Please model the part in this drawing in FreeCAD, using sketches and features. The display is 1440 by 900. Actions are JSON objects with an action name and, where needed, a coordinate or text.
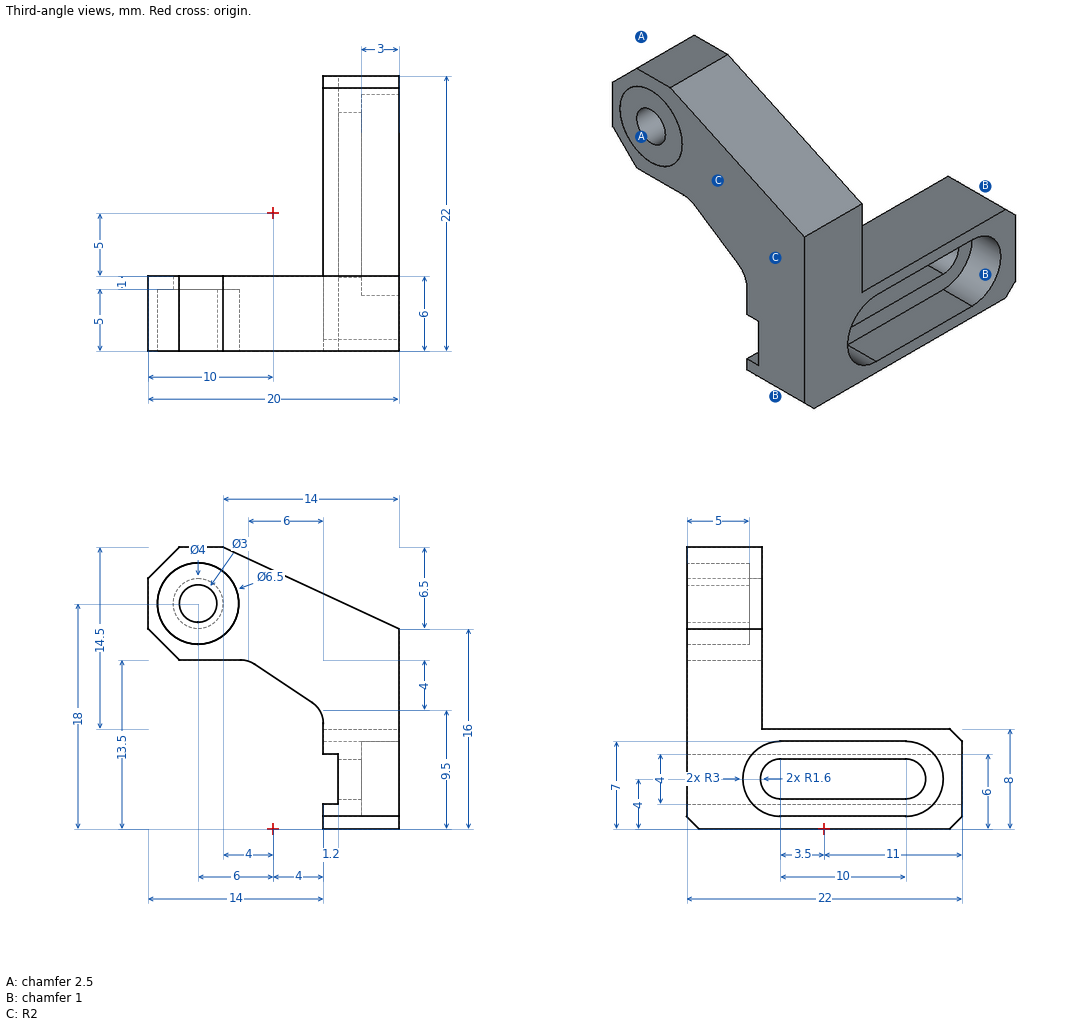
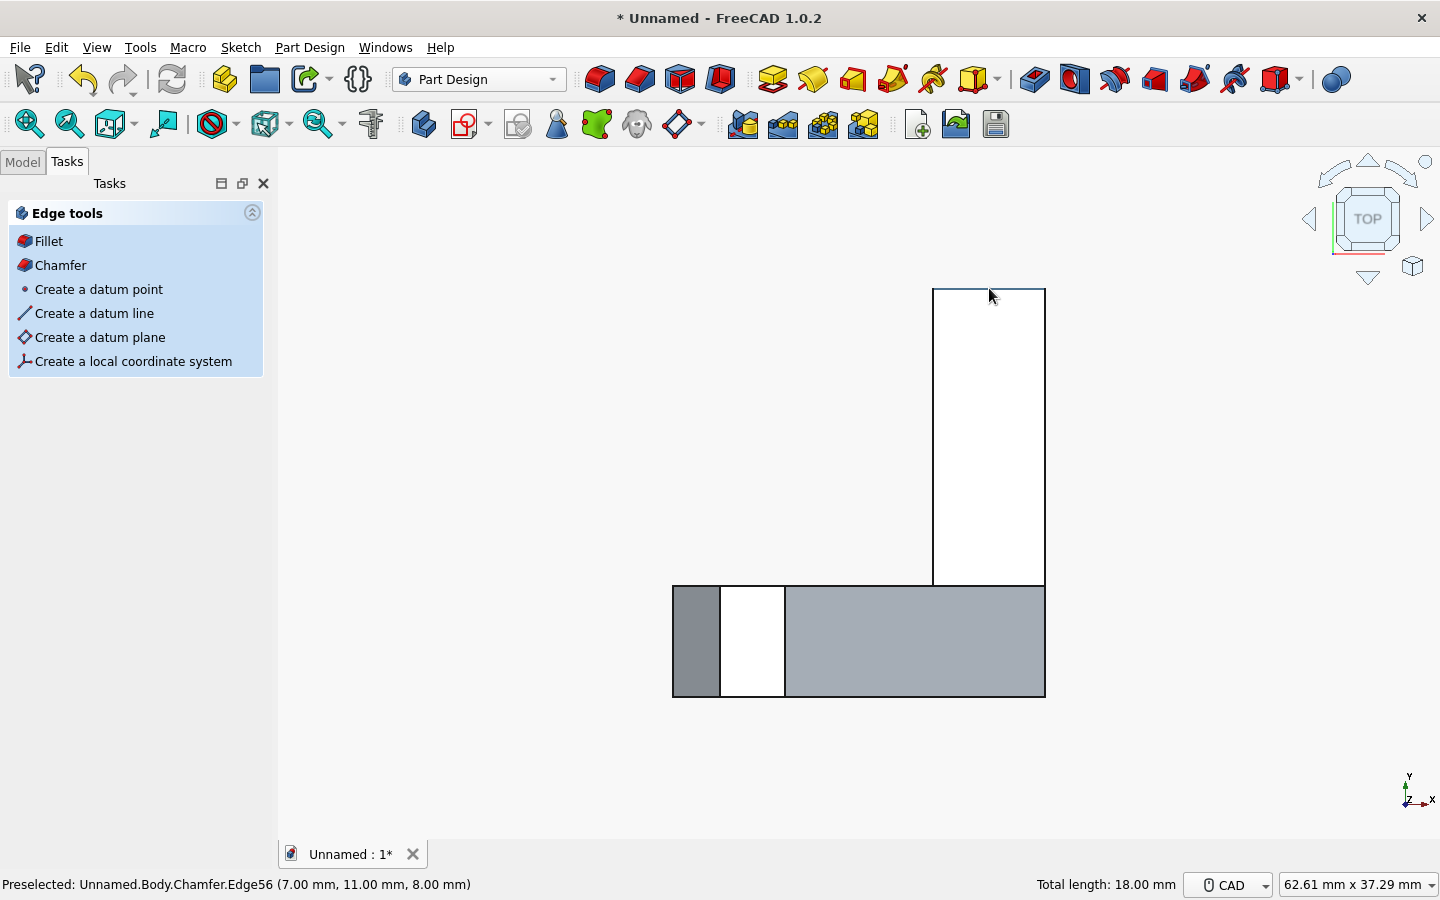
{"action": "left_click", "coordinate": [640, 80]}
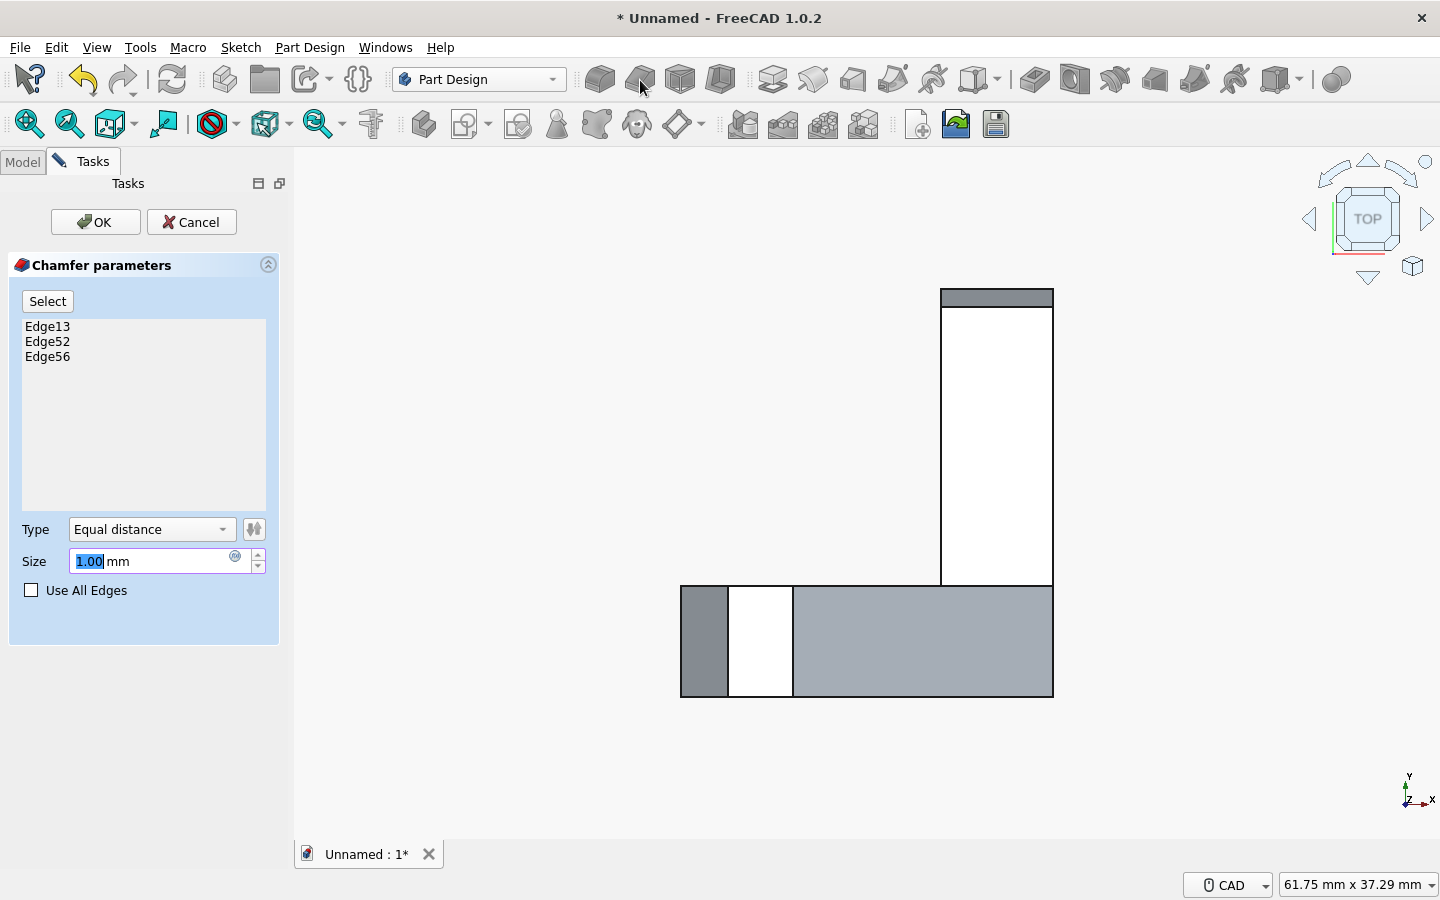
{"action": "type", "text": "1"}
{"action": "key", "text": "Tab"}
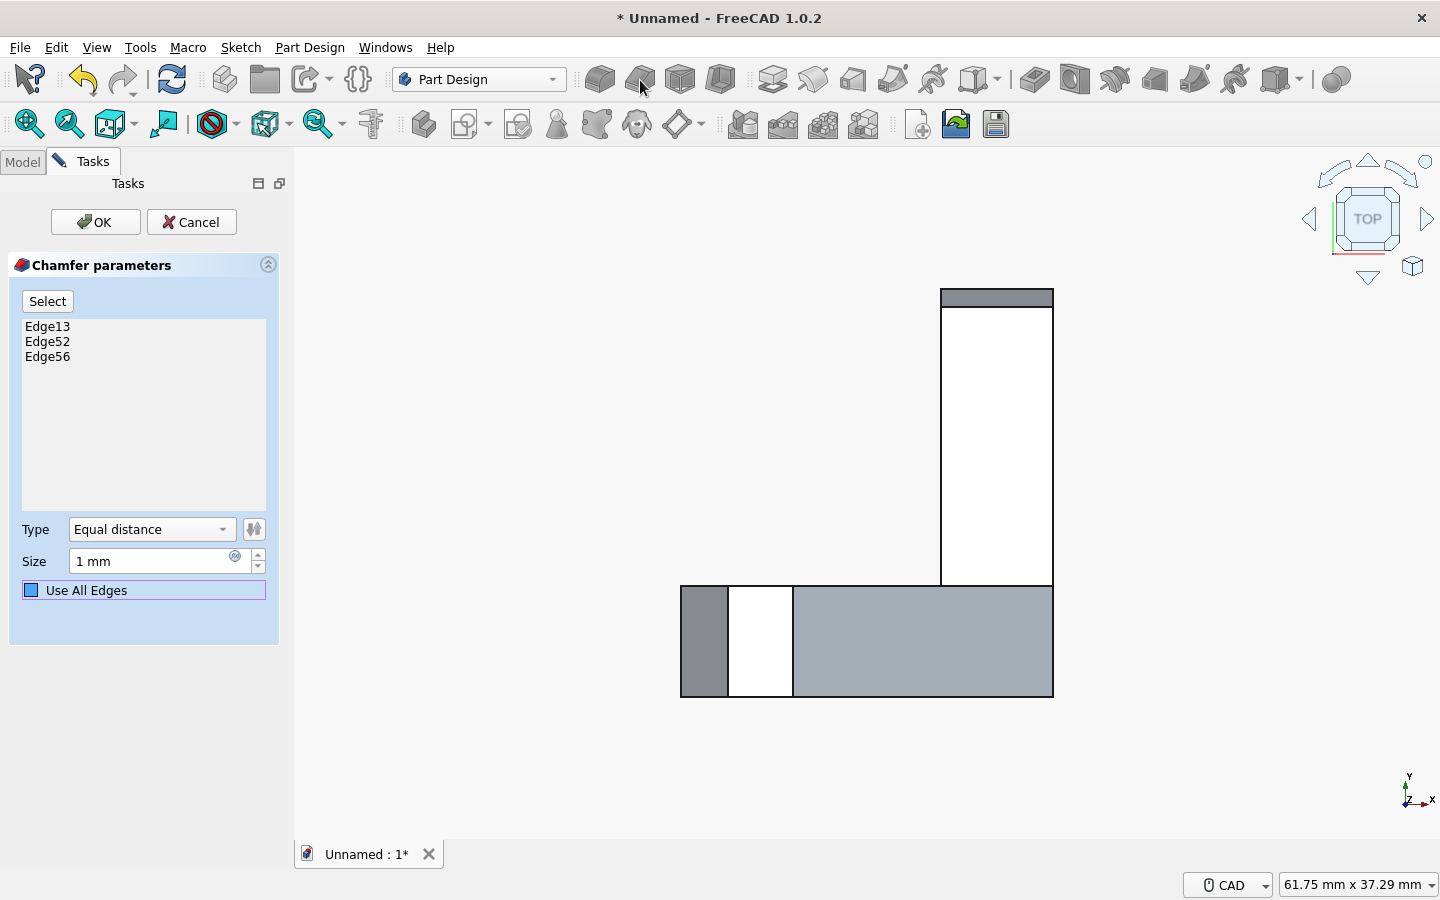
{"action": "left_click", "coordinate": [96, 222]}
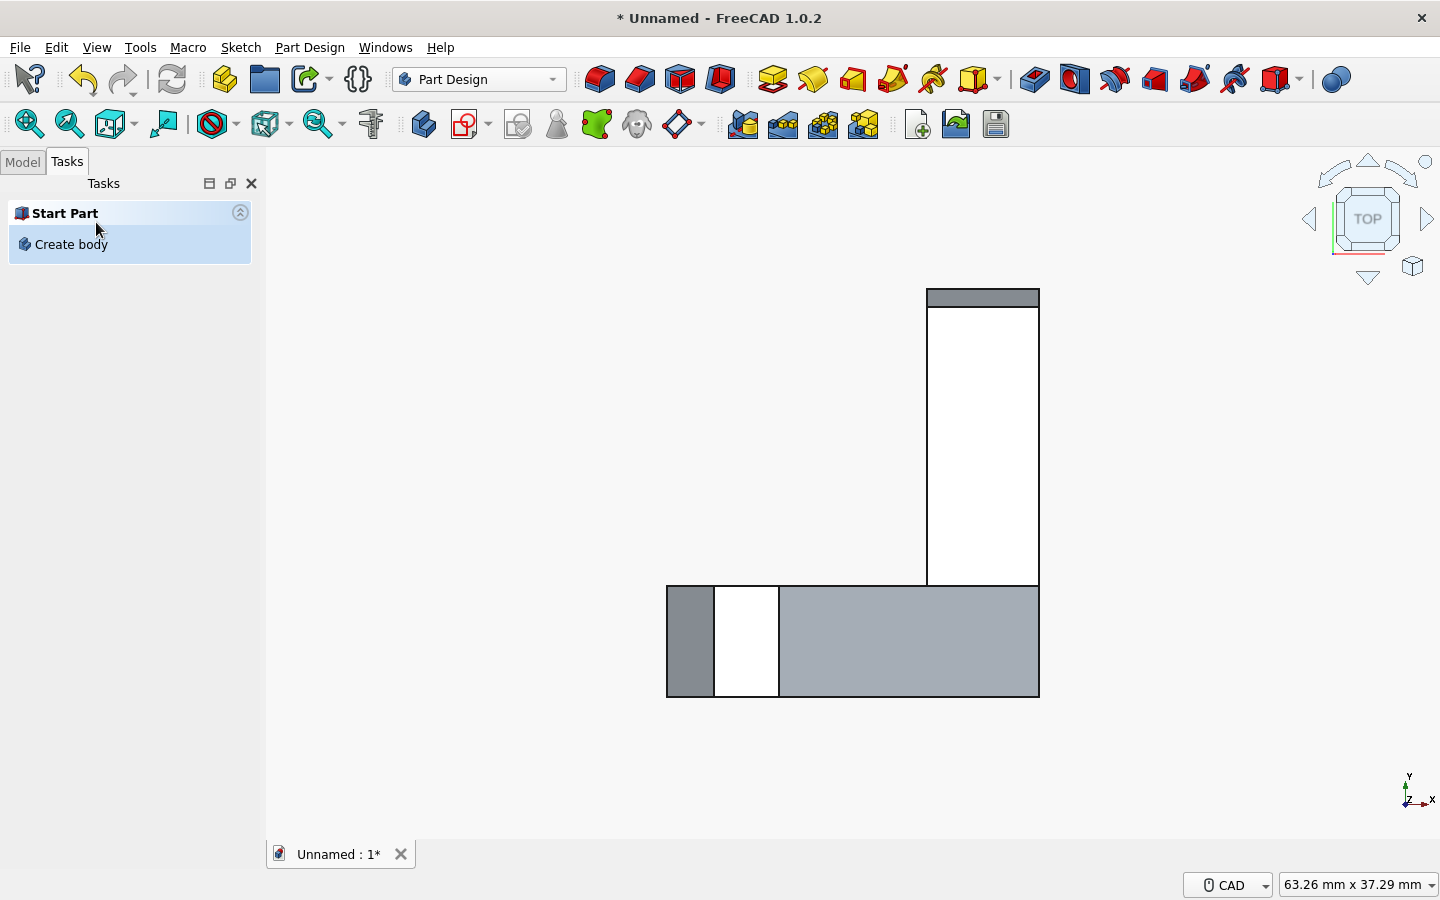
{"action": "key", "text": "0"}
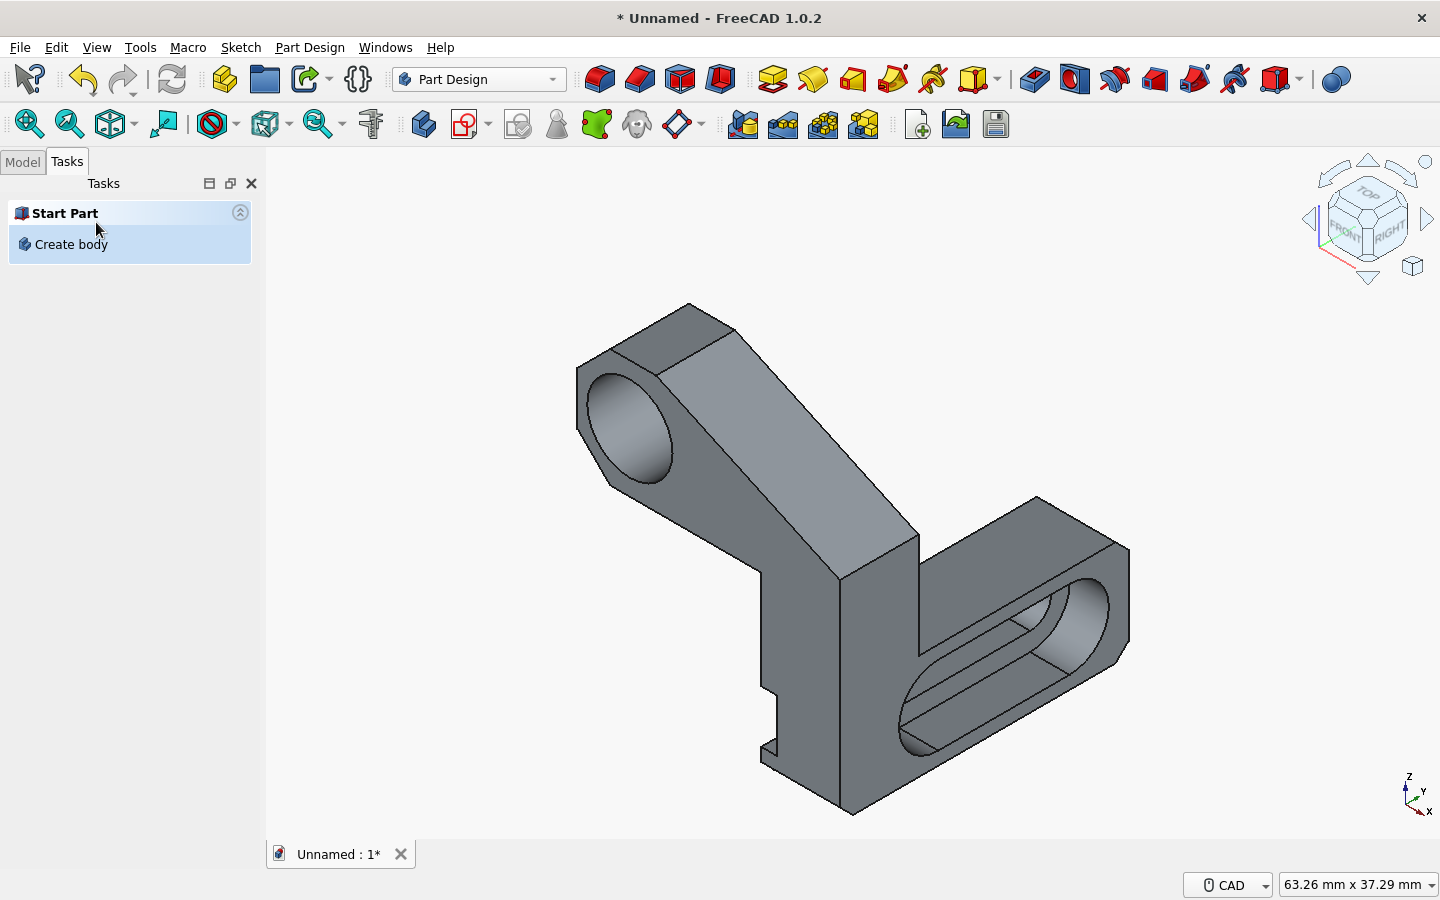
{"action": "left_click", "coordinate": [709, 475]}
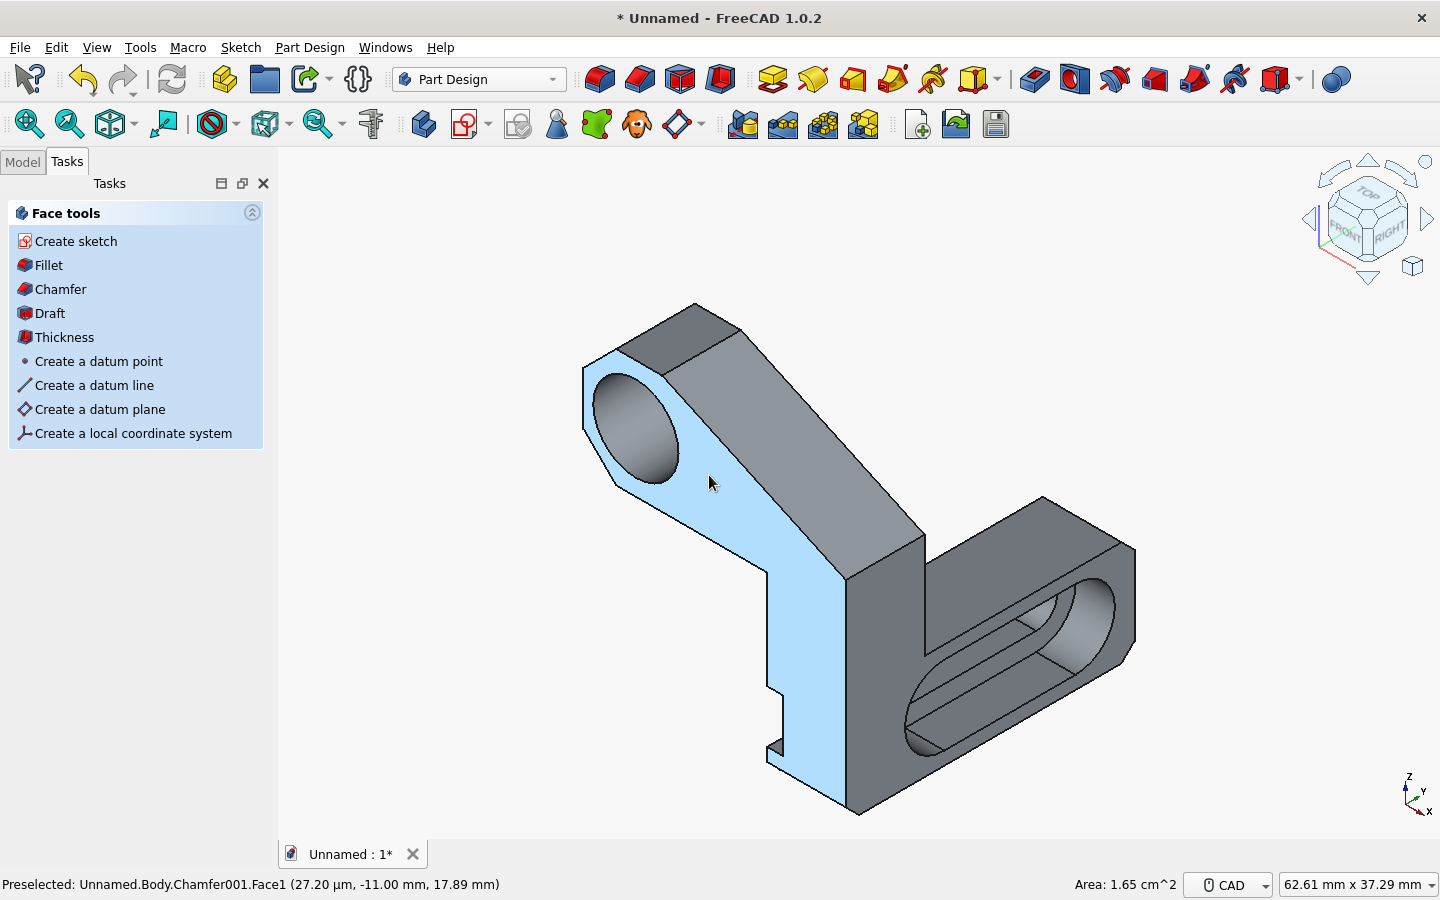
{"action": "left_click", "coordinate": [464, 124]}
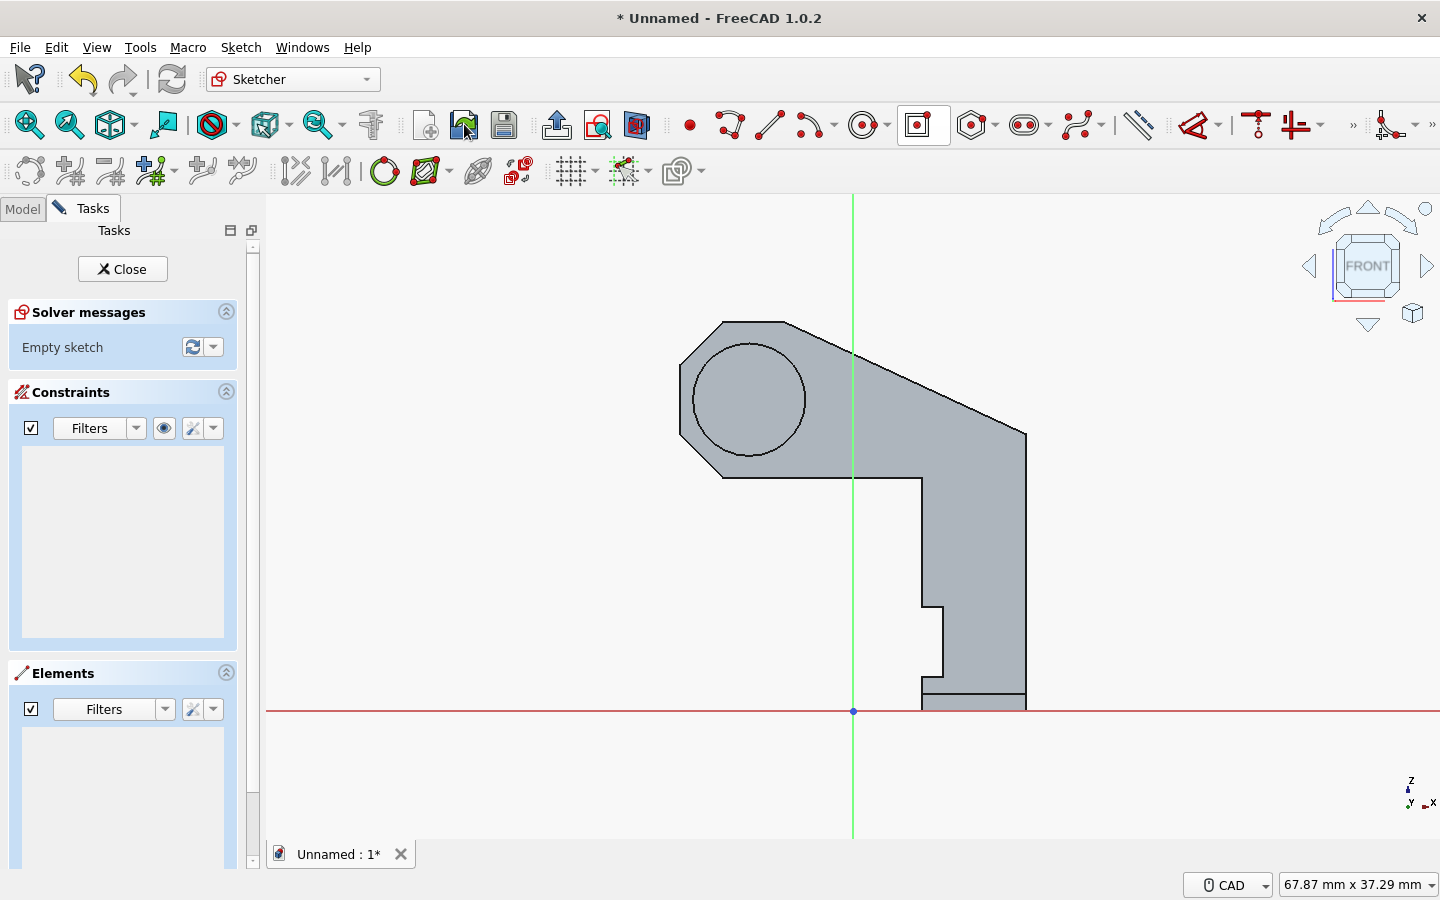
{"action": "scroll", "coordinate": [975, 689], "scroll_direction": "up", "scroll_amount": 3}